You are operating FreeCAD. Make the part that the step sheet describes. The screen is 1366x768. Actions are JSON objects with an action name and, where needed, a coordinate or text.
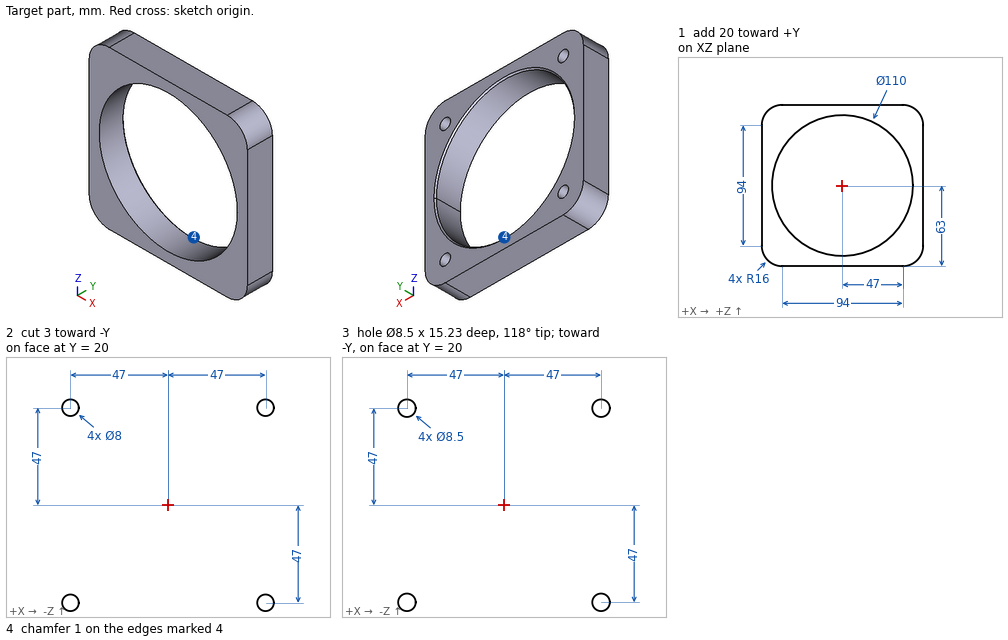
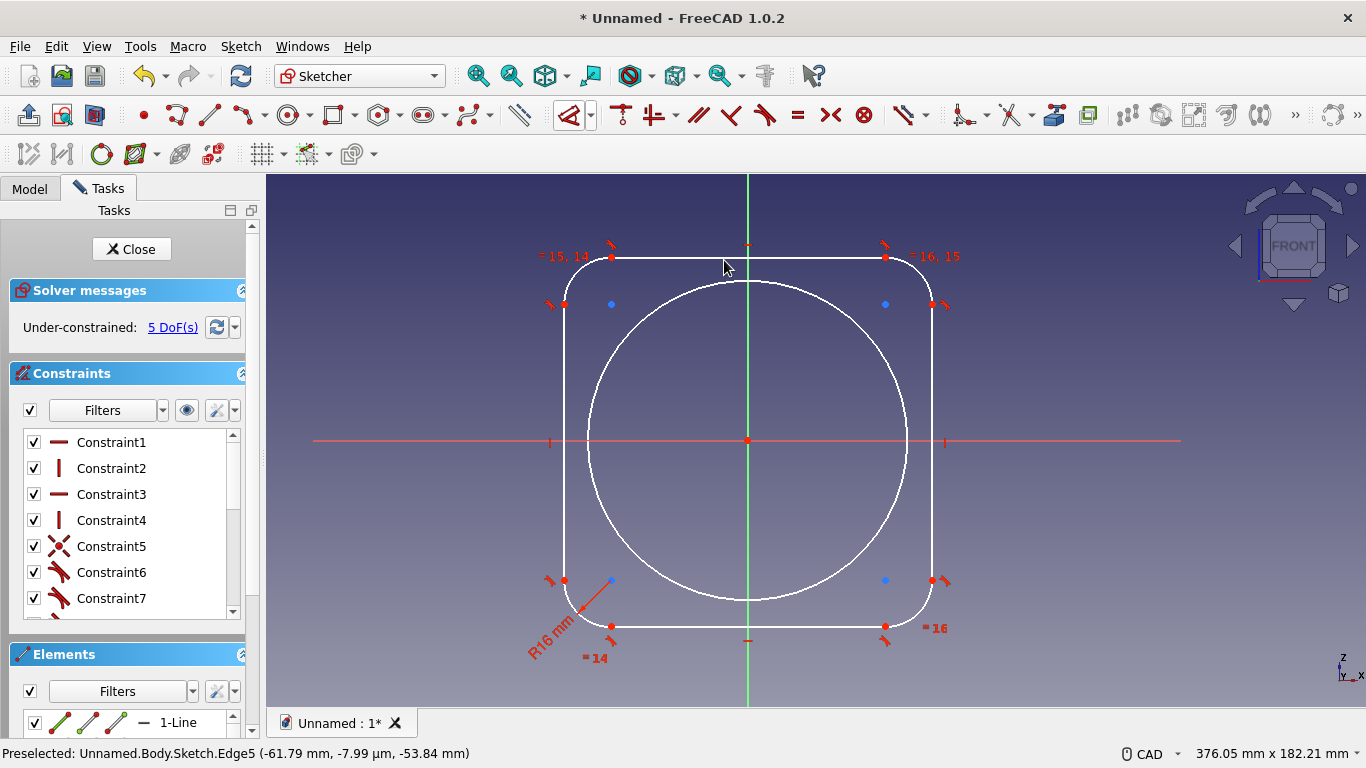
{"action": "left_click", "coordinate": [860, 327]}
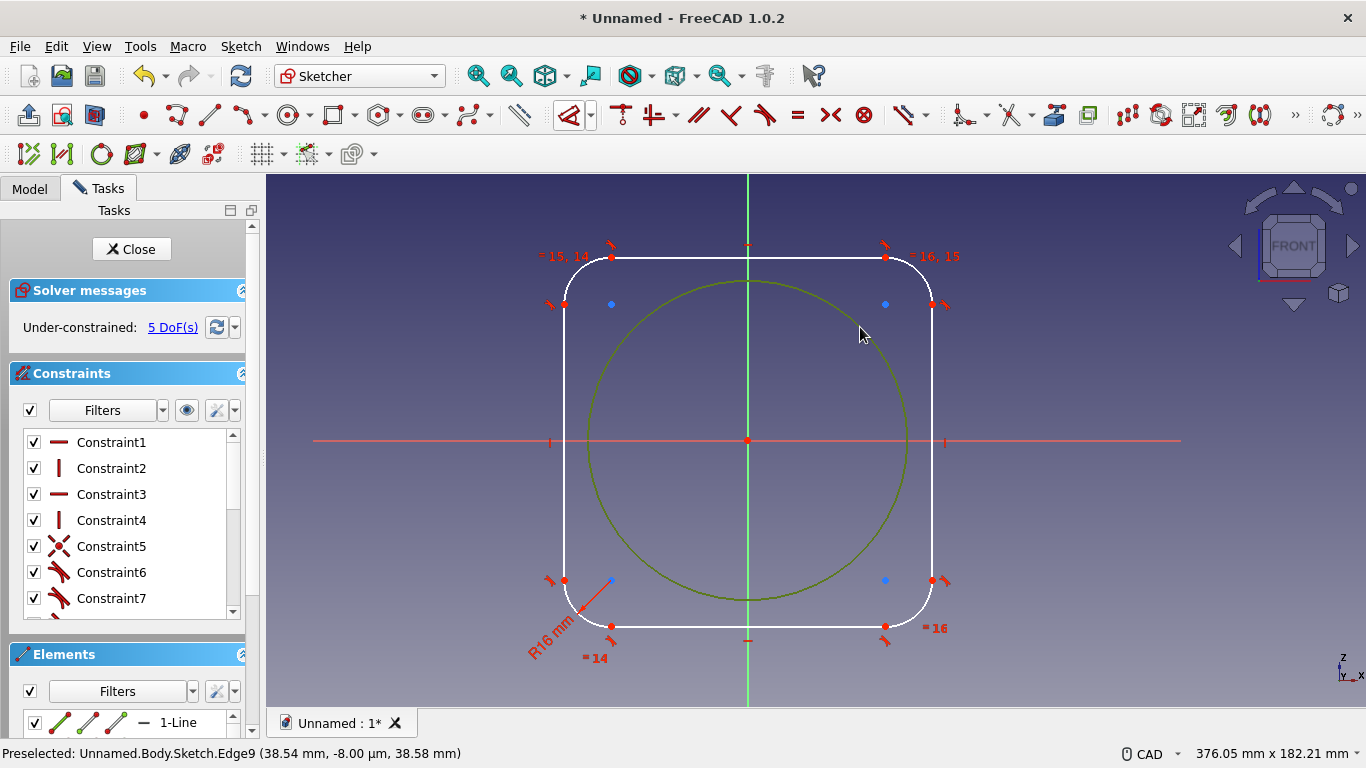
{"action": "left_click", "coordinate": [590, 116]}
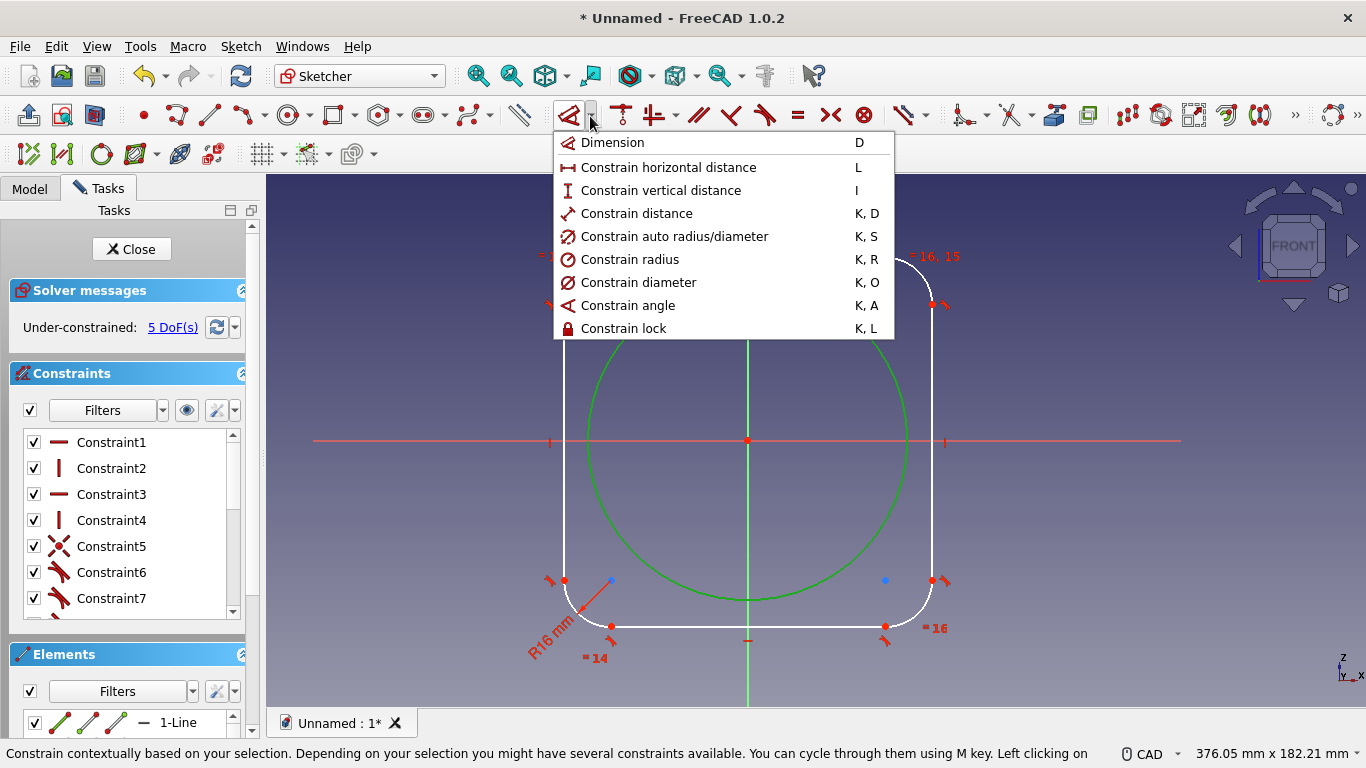
{"action": "left_click", "coordinate": [724, 282]}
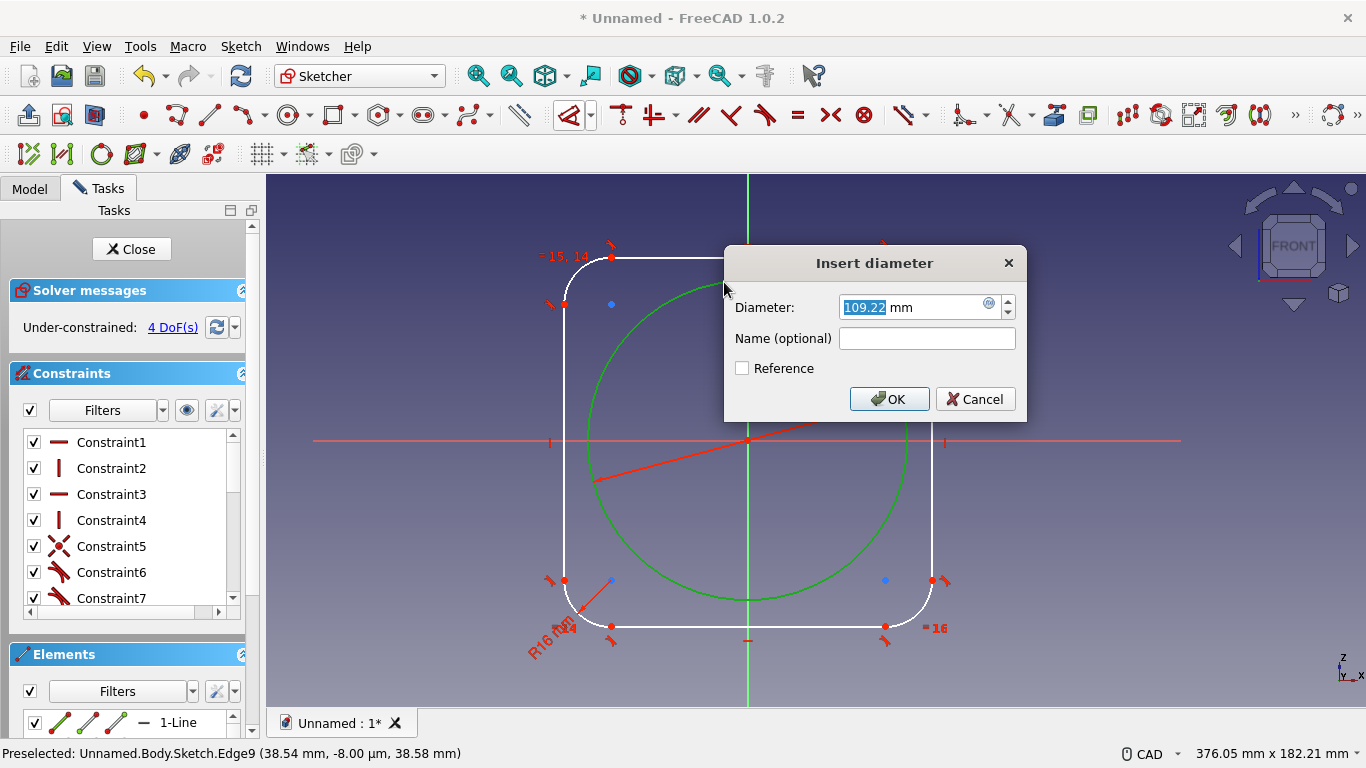
{"action": "type", "text": "110"}
{"action": "key", "text": "Return"}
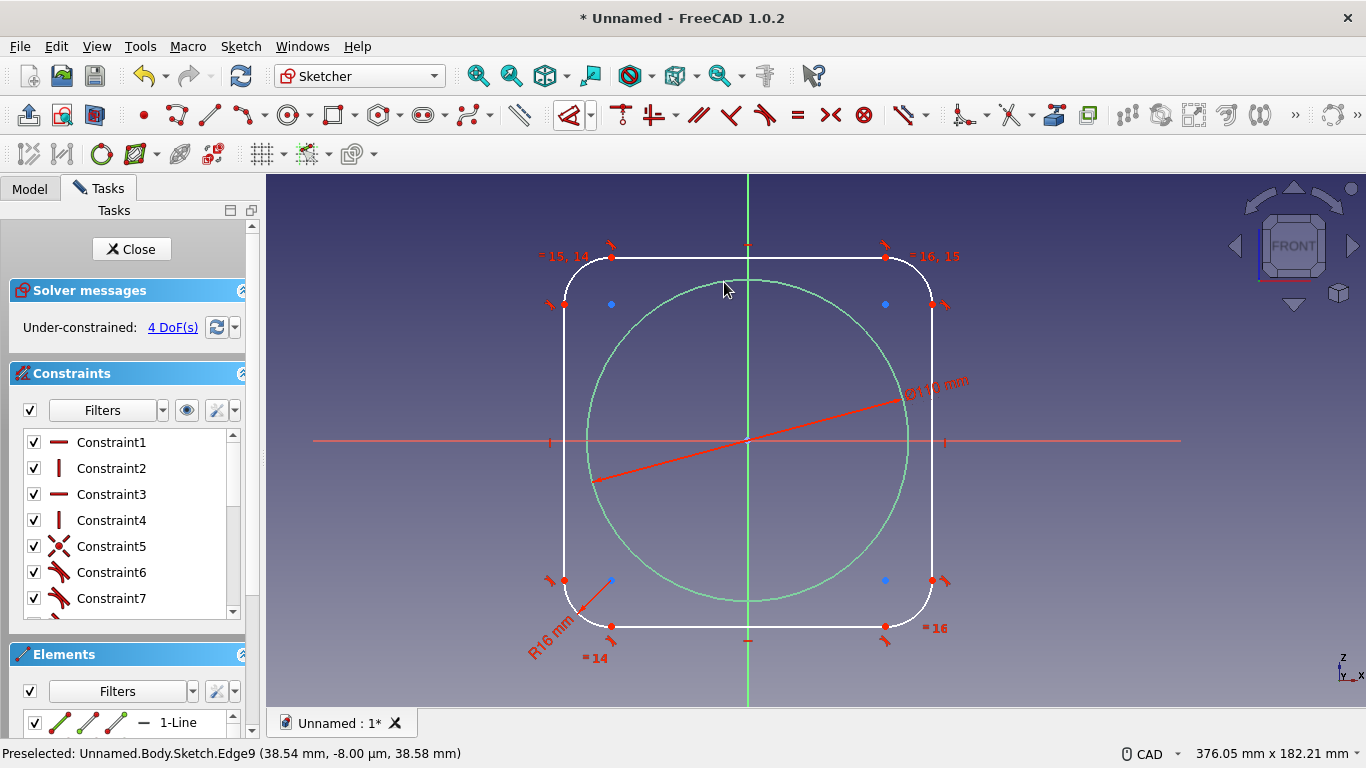
{"action": "left_click", "coordinate": [803, 627]}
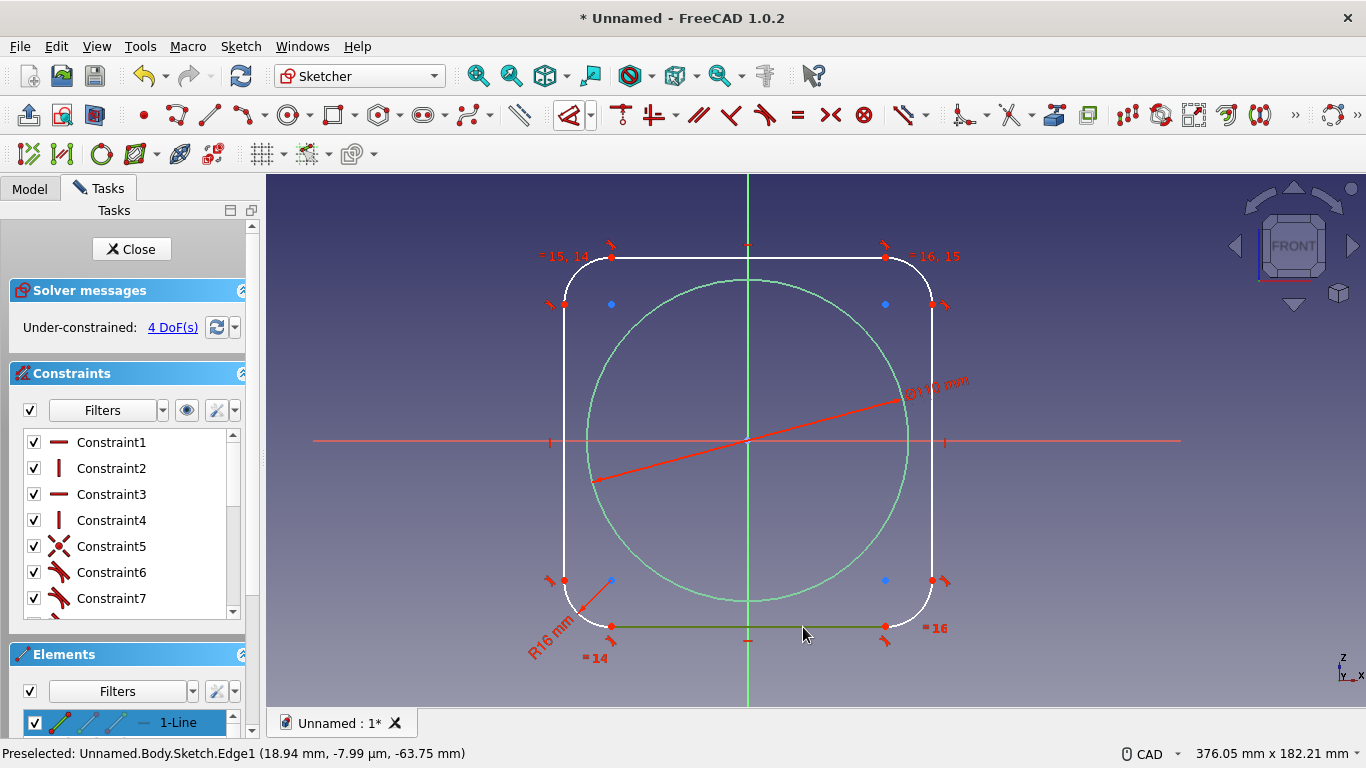
{"action": "left_click", "coordinate": [590, 116]}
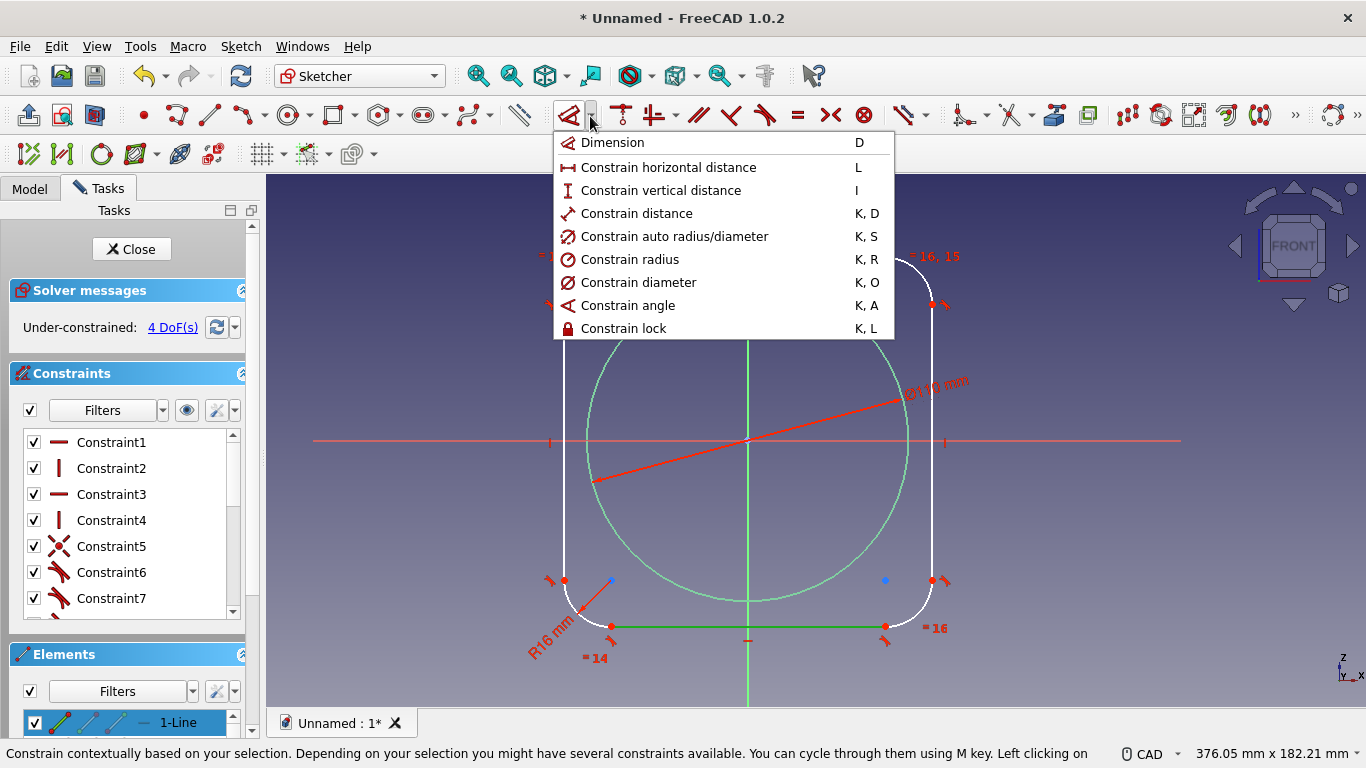
{"action": "left_click", "coordinate": [724, 168]}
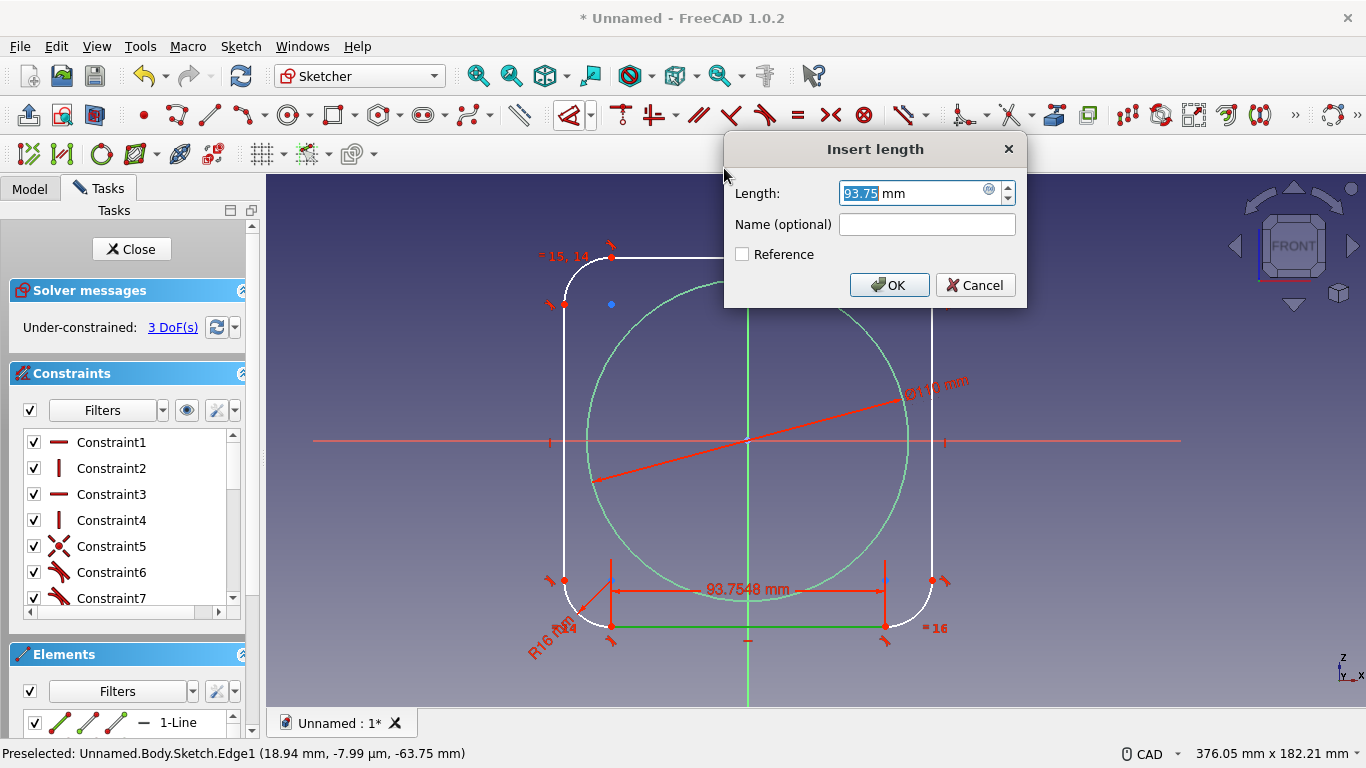
{"action": "type", "text": "94"}
{"action": "key", "text": "Return"}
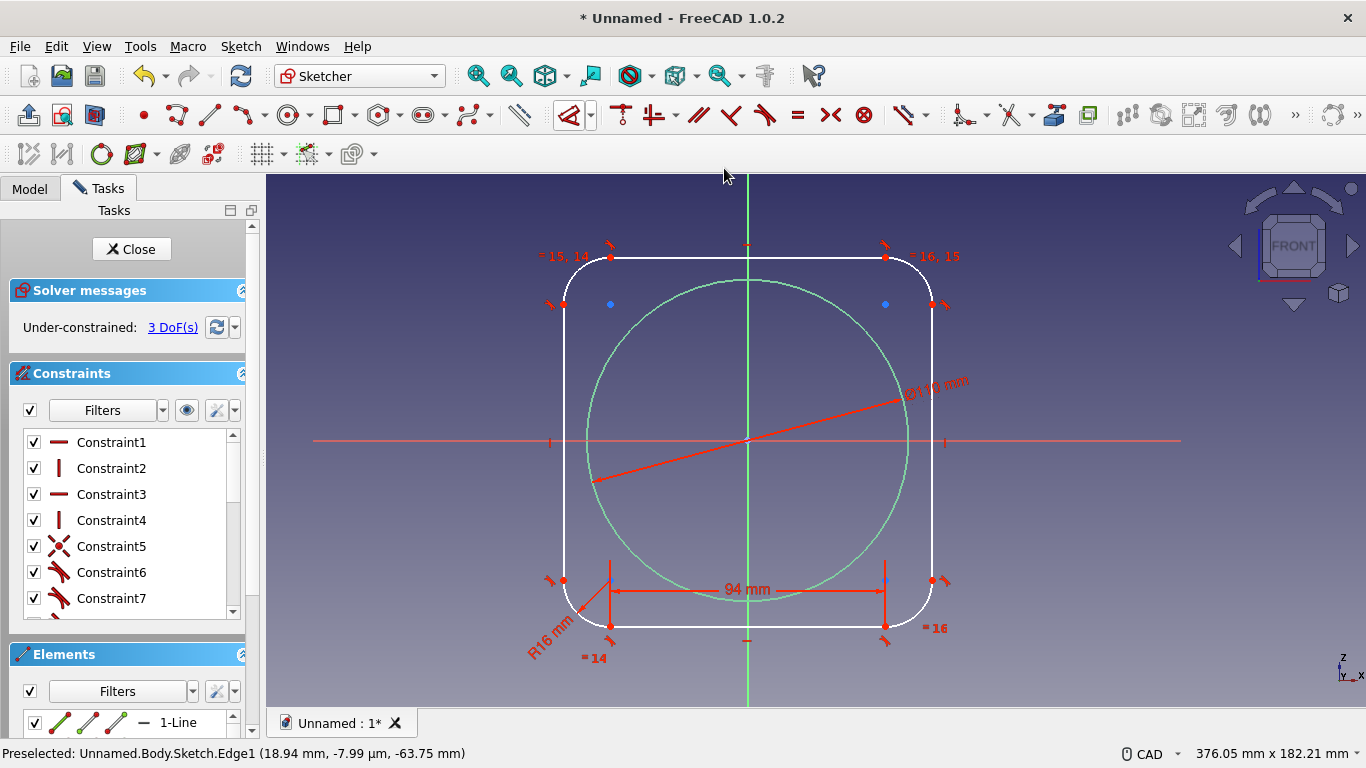
{"action": "left_click", "coordinate": [564, 497]}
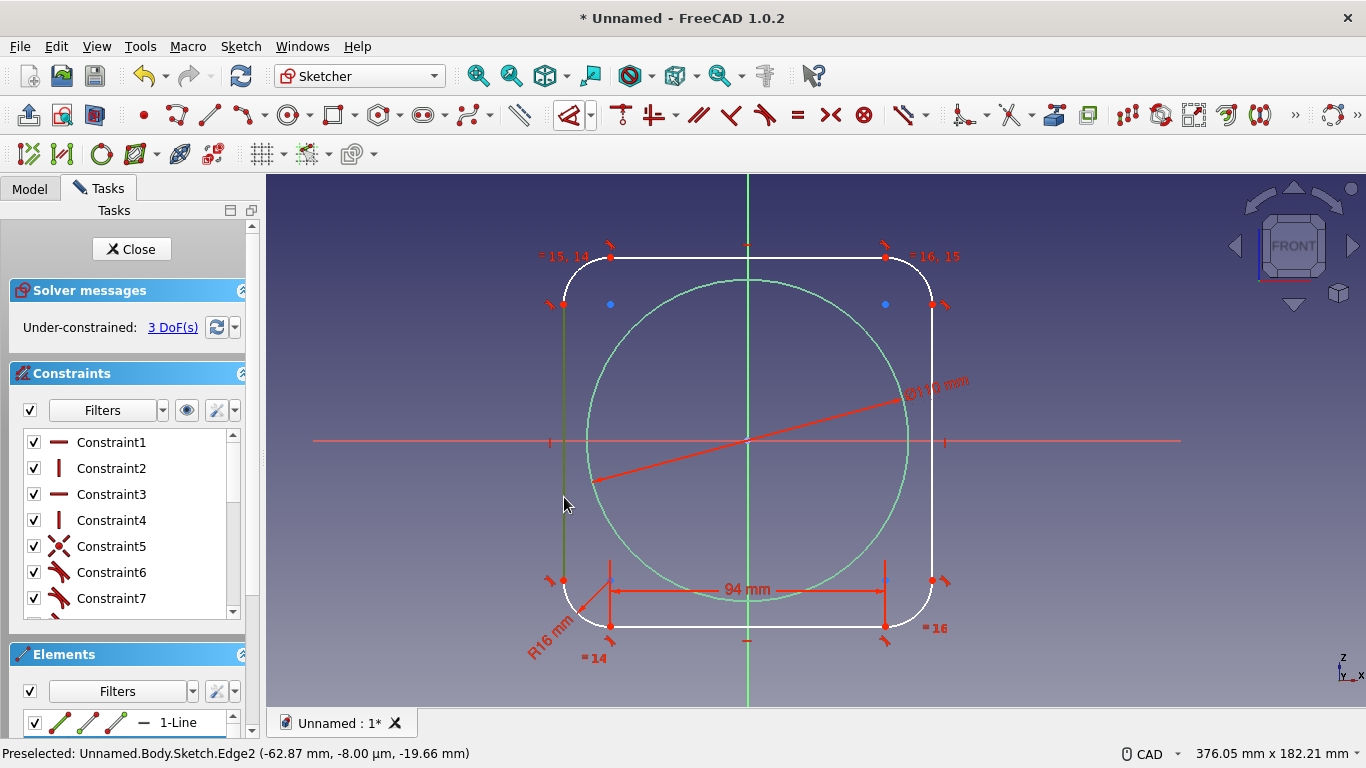
{"action": "left_click", "coordinate": [590, 116]}